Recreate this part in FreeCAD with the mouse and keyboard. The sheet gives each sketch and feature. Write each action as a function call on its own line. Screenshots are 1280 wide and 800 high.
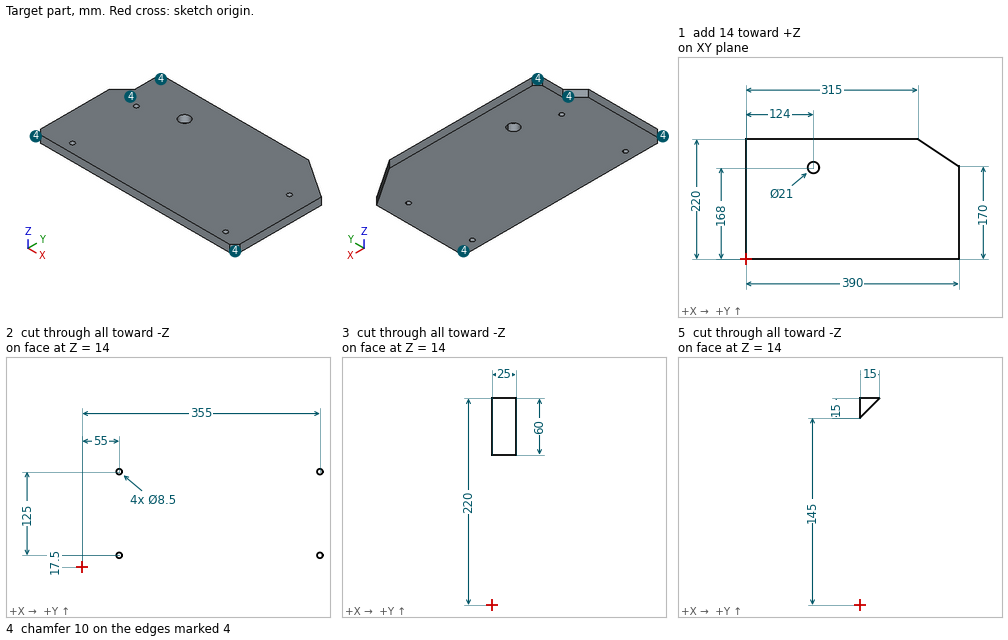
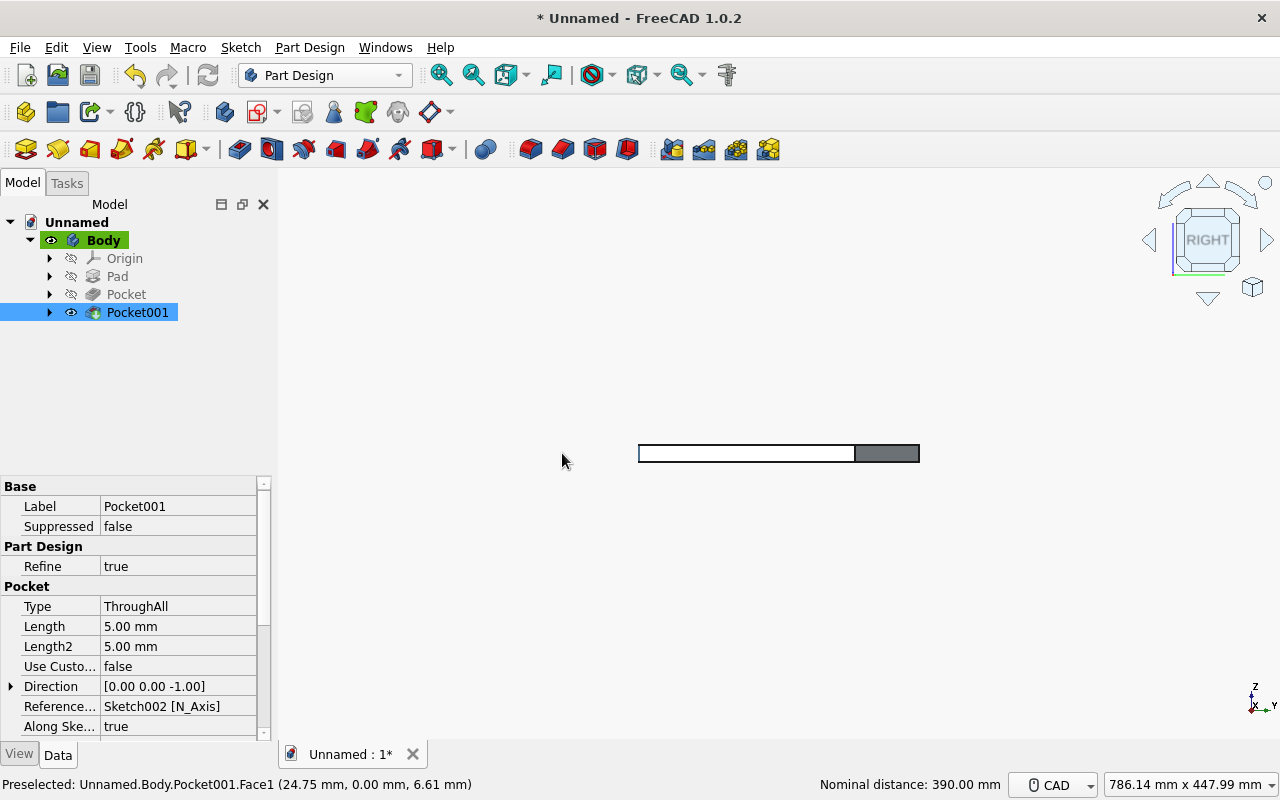
scroll(919, 452, up, 5)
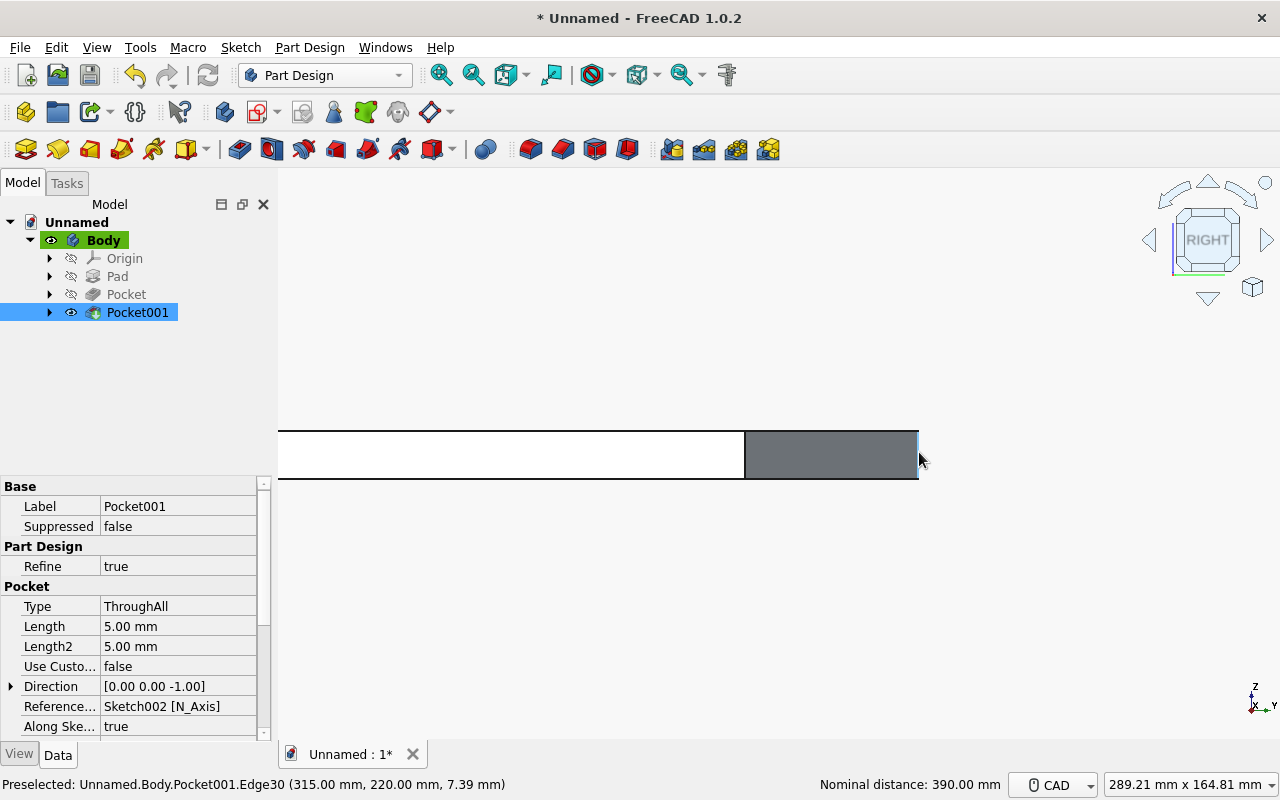
key(v)
key(f)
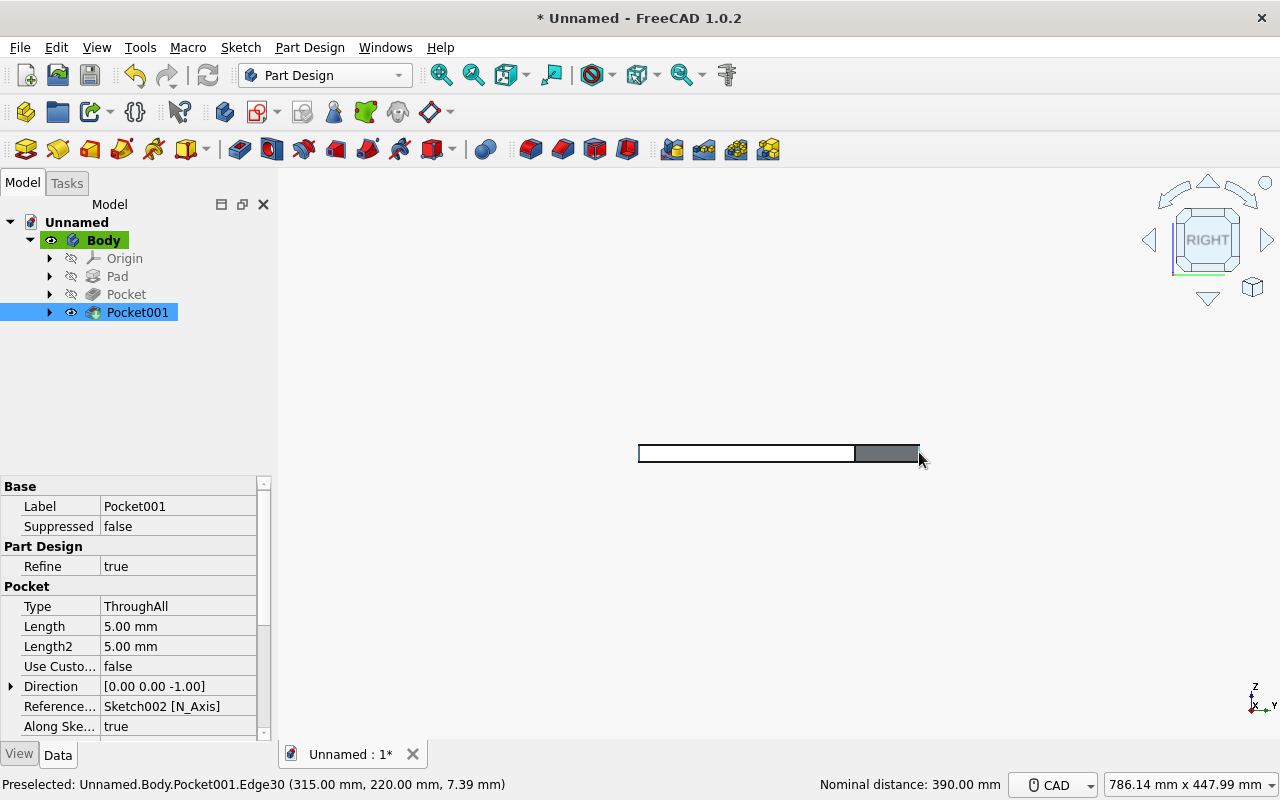
key(5)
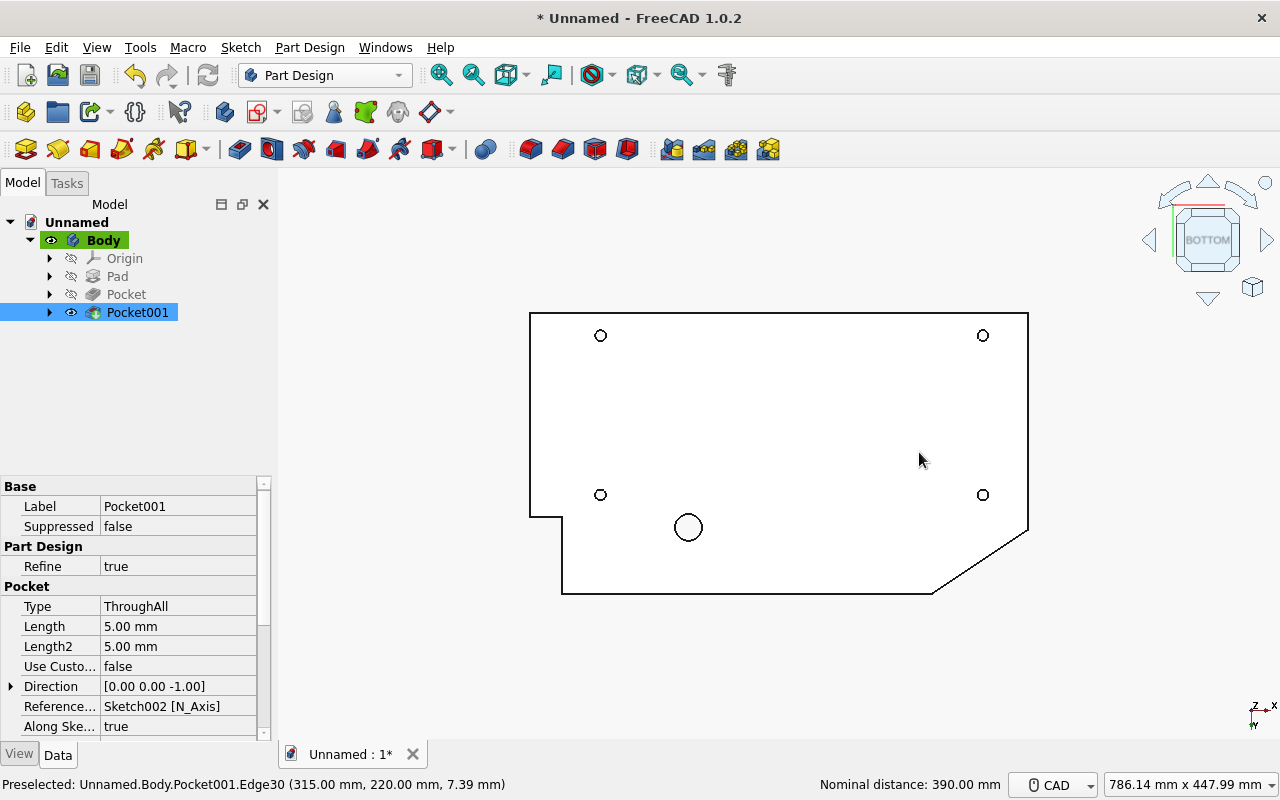
scroll(562, 593, up, 5)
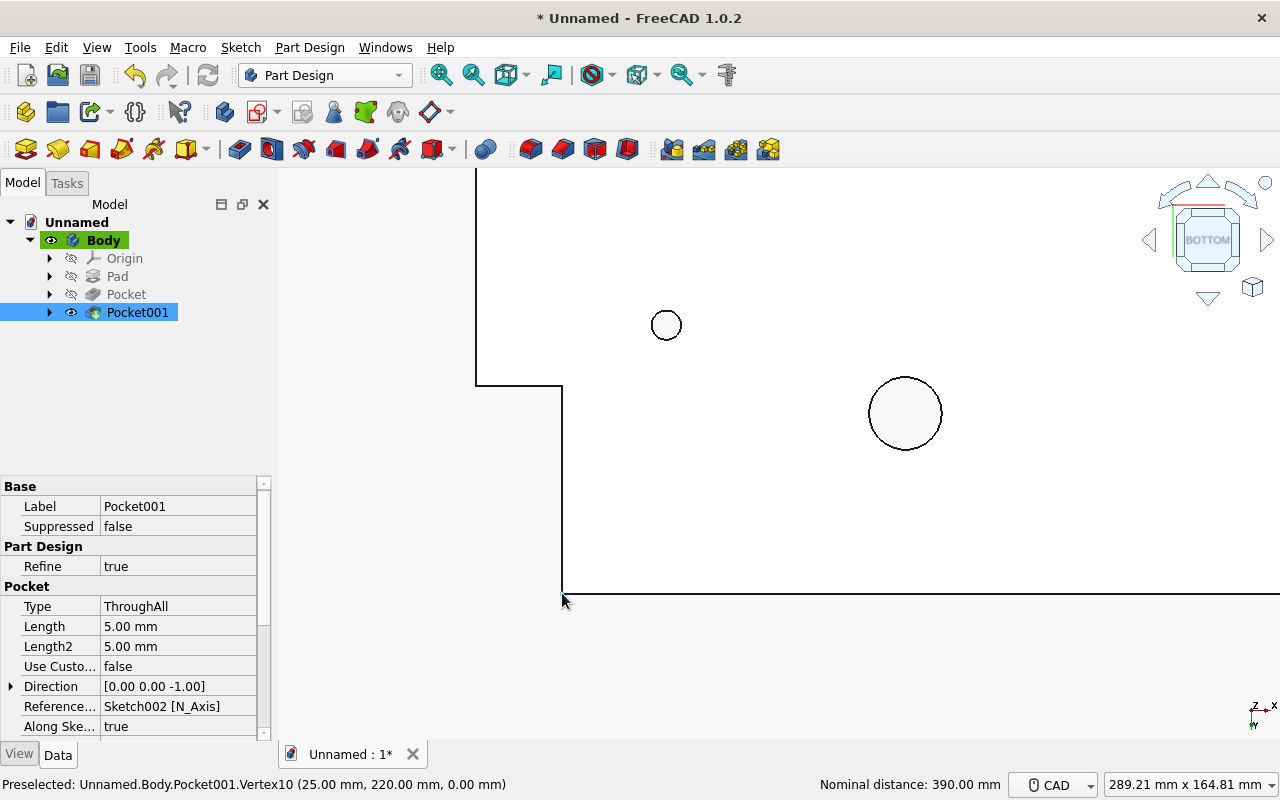
key(v)
key(f)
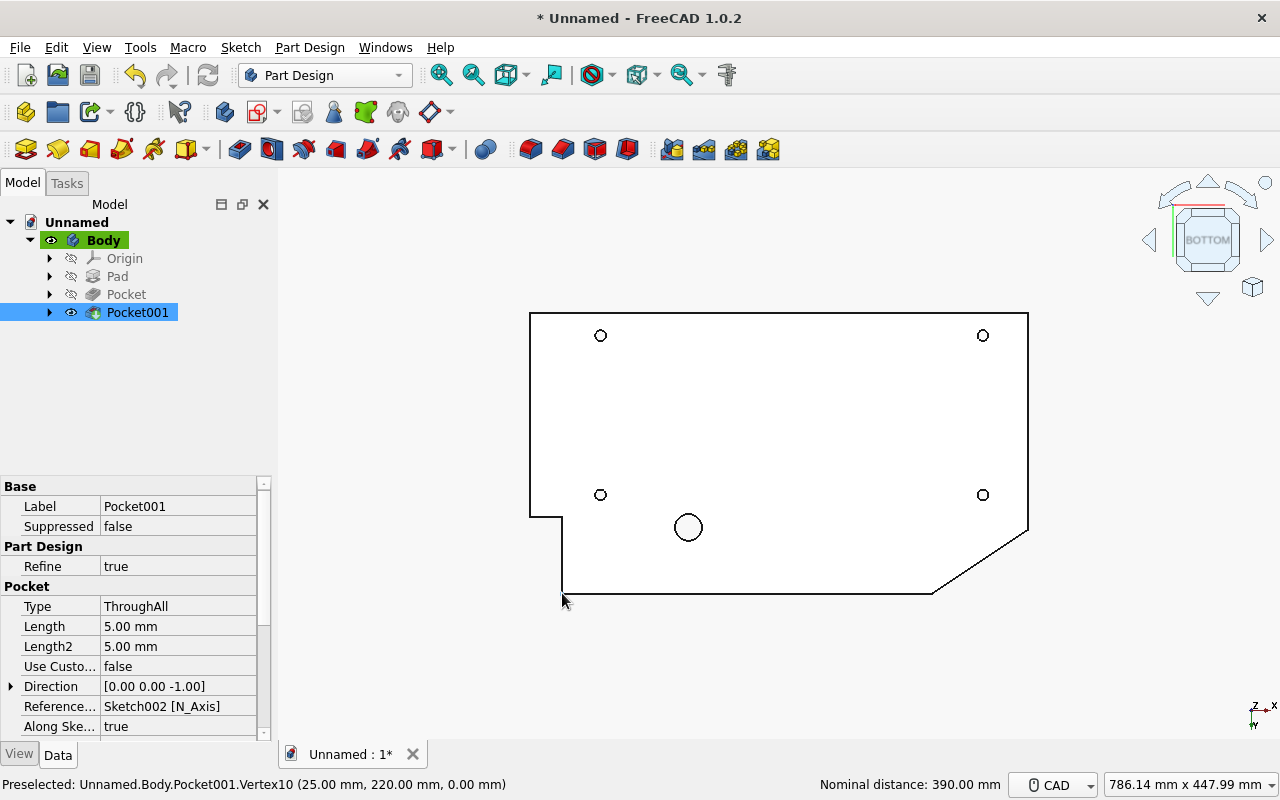
key(4)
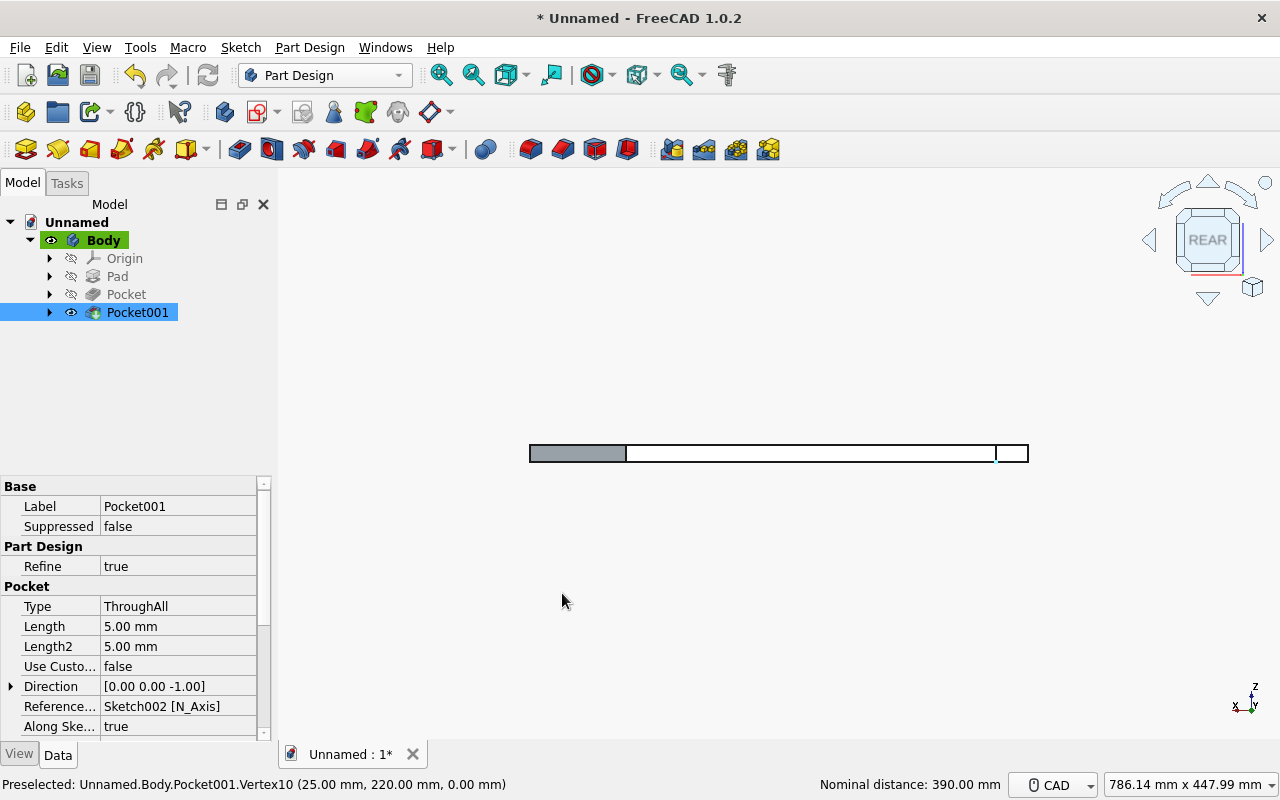
click(996, 453, ctrl)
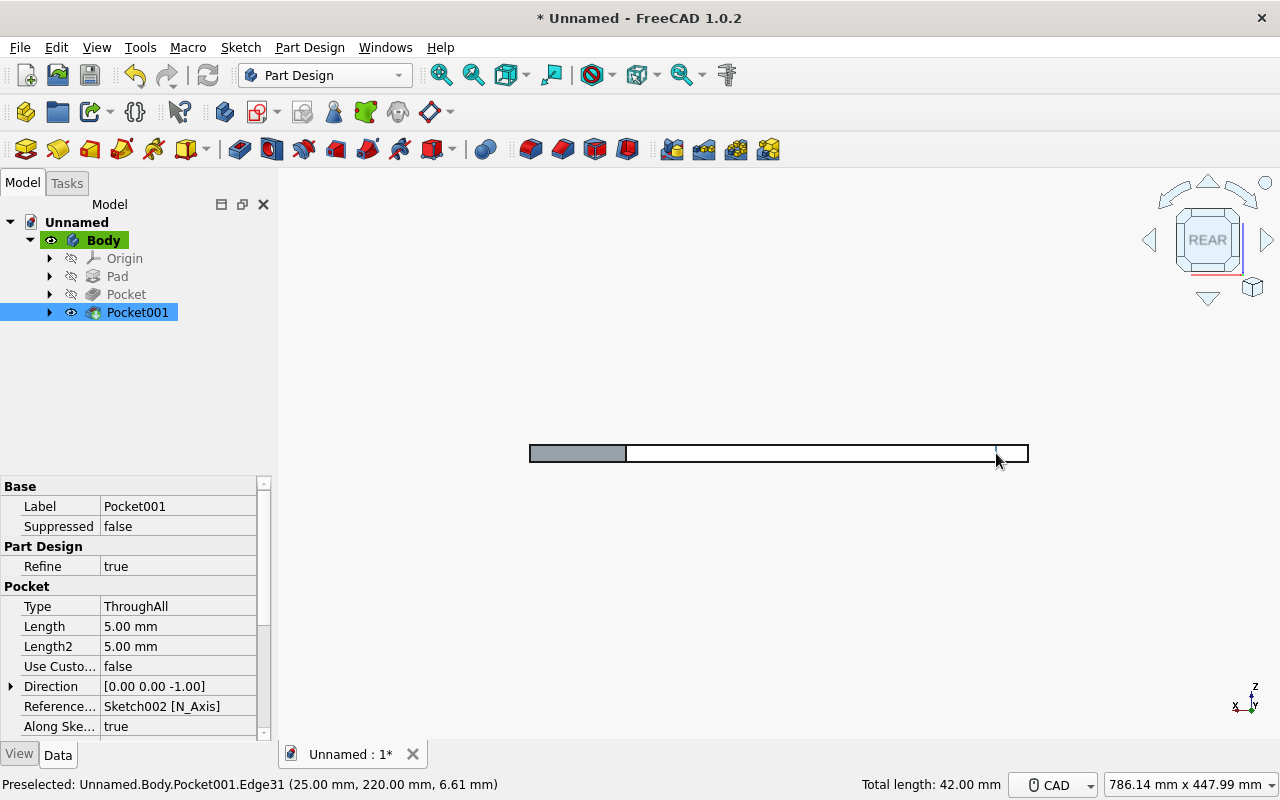
scroll(996, 453, up, 5)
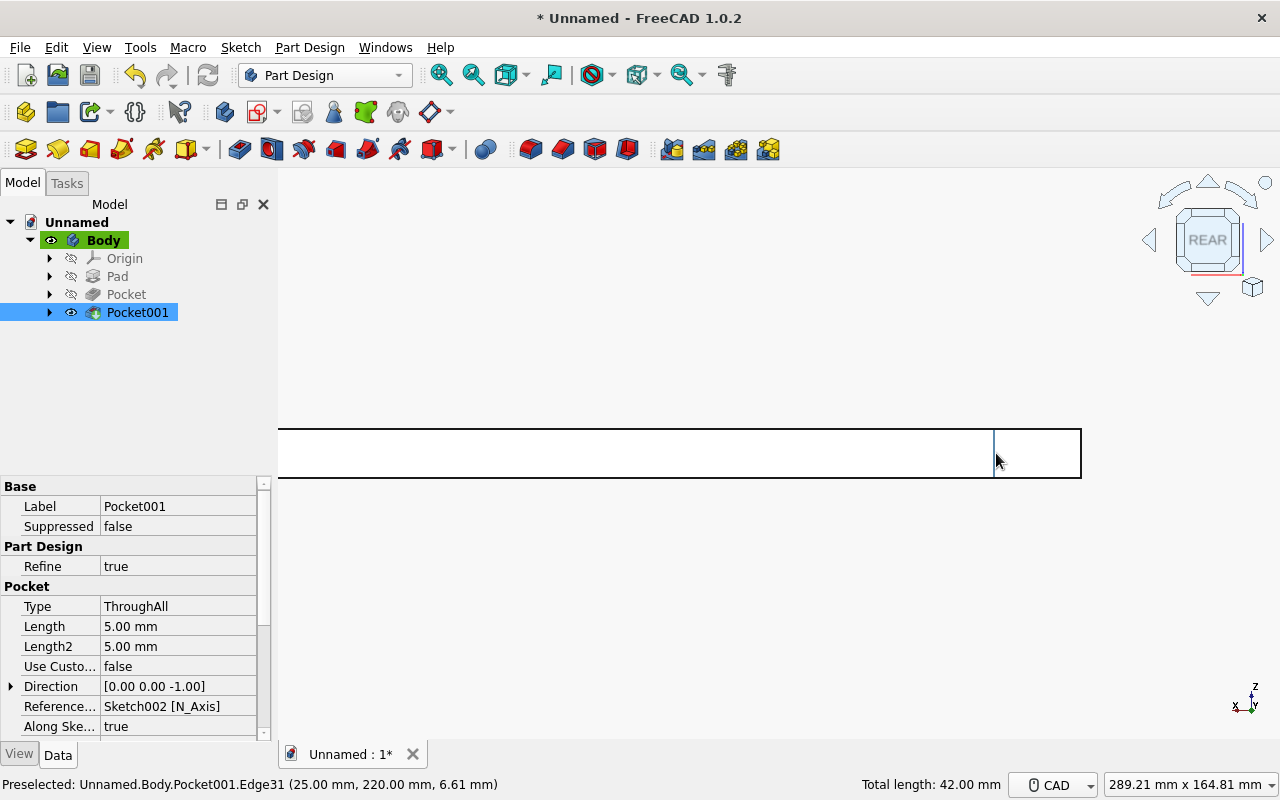
key(v)
key(f)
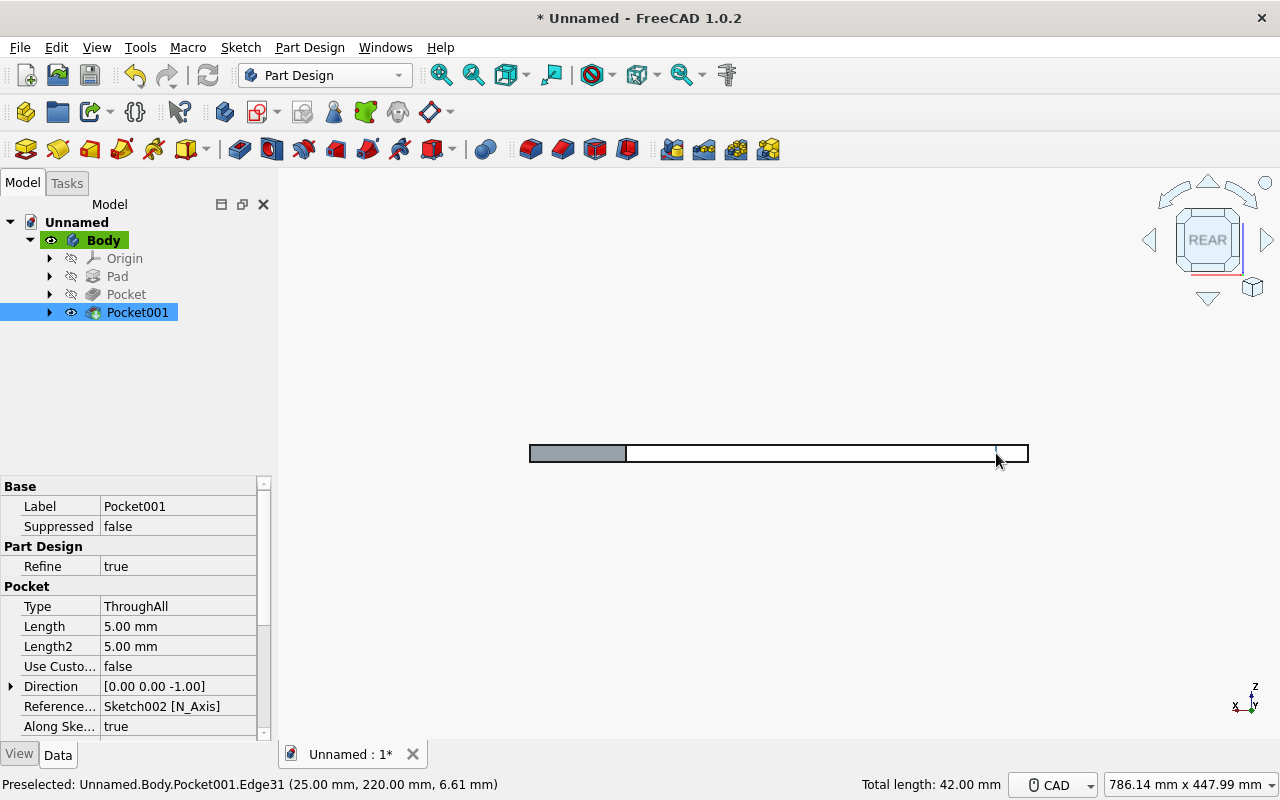
key(6)